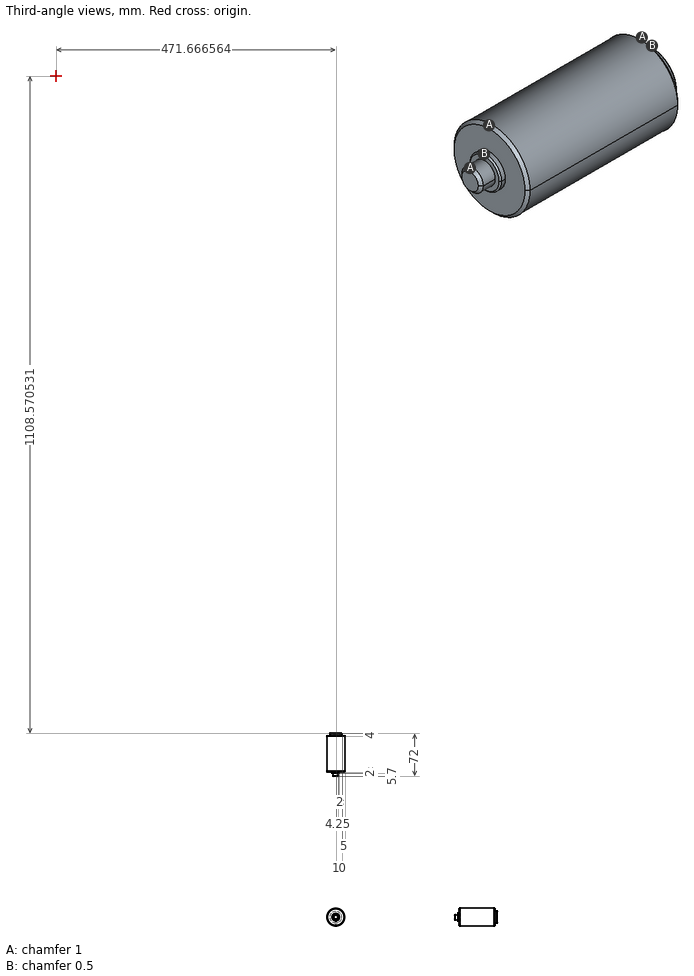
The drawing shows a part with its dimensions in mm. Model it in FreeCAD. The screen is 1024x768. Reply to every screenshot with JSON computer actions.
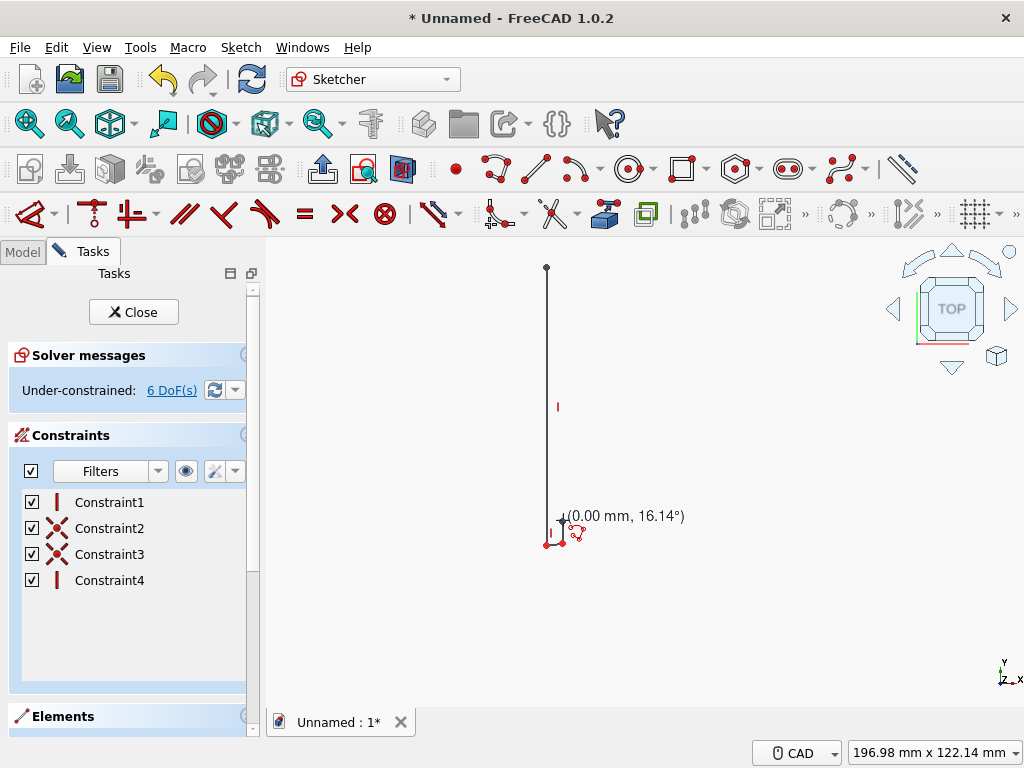
{"action": "scroll", "coordinate": [571, 520], "scroll_direction": "up", "scroll_amount": 4}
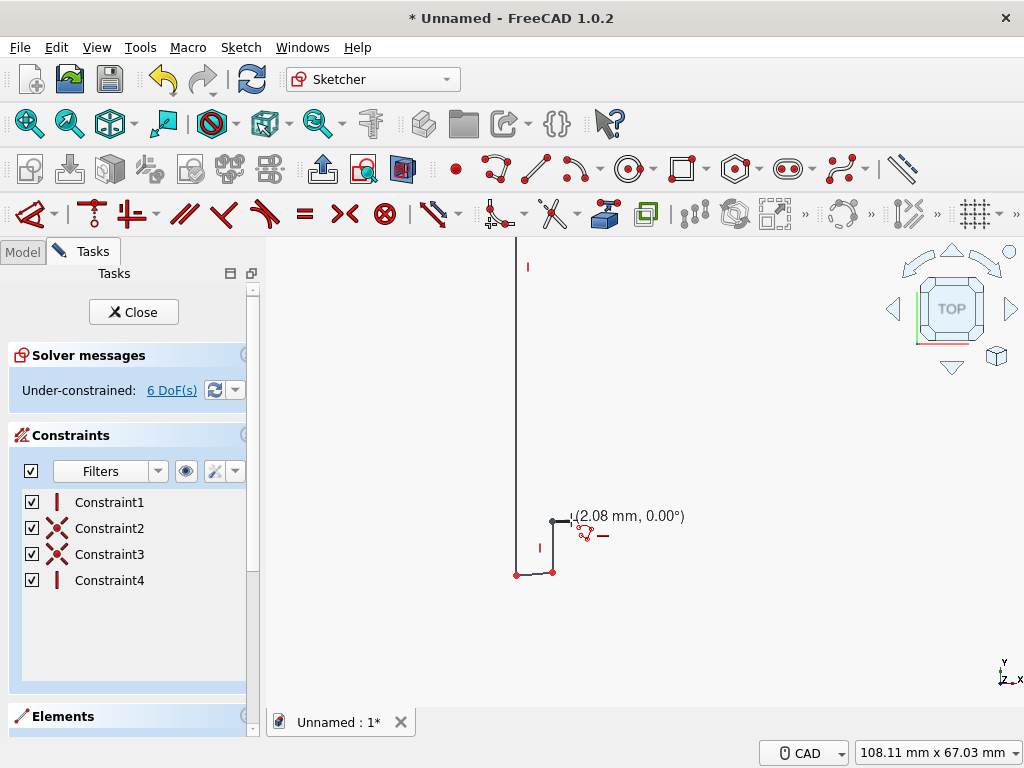
{"action": "left_click", "coordinate": [571, 519]}
{"action": "left_click", "coordinate": [571, 503]}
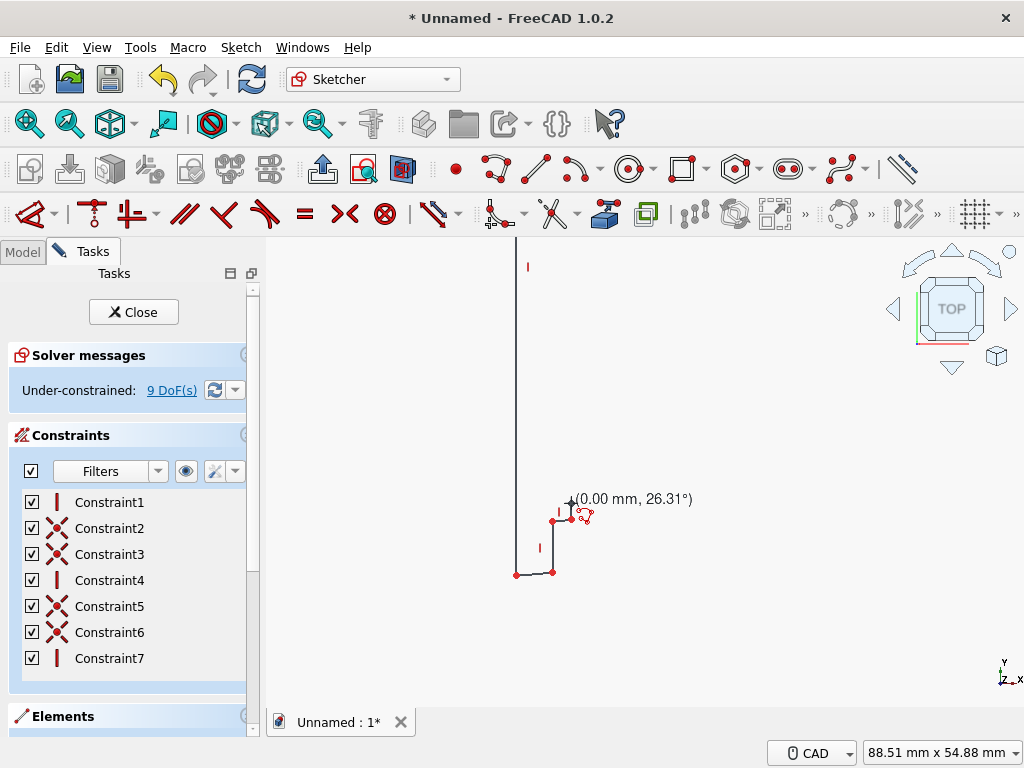
{"action": "scroll", "coordinate": [574, 667], "scroll_direction": "down", "scroll_amount": 5}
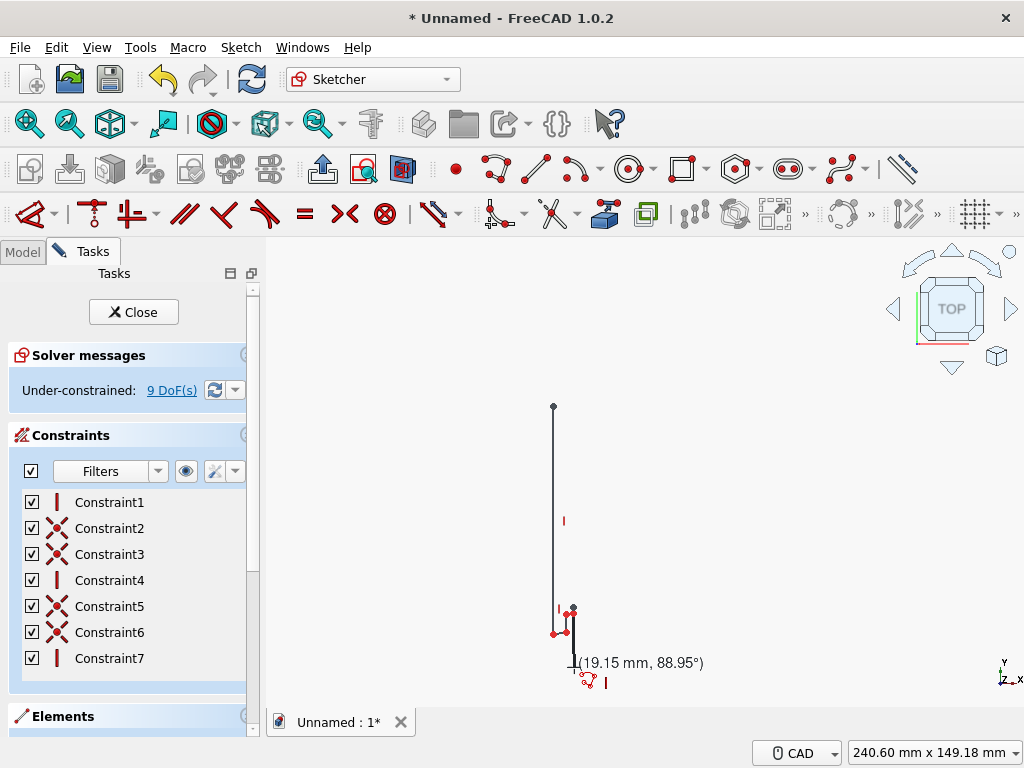
{"action": "left_click", "coordinate": [601, 607]}
{"action": "left_click", "coordinate": [601, 417]}
{"action": "left_click", "coordinate": [585, 417]}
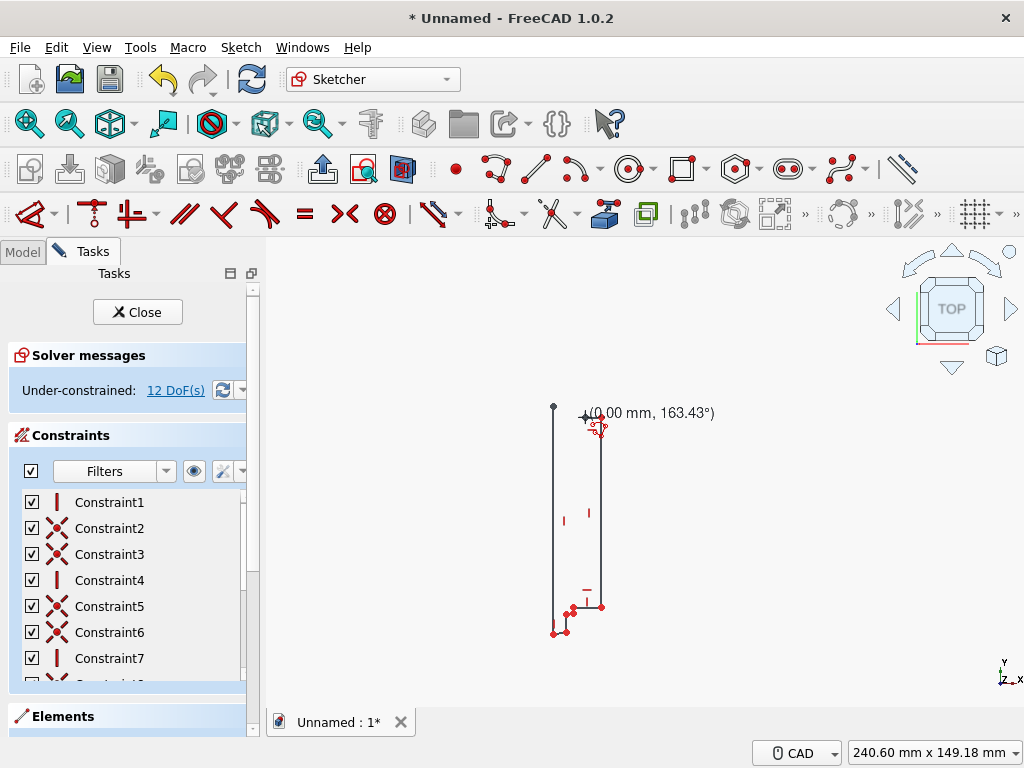
{"action": "scroll", "coordinate": [585, 405], "scroll_direction": "up", "scroll_amount": 2}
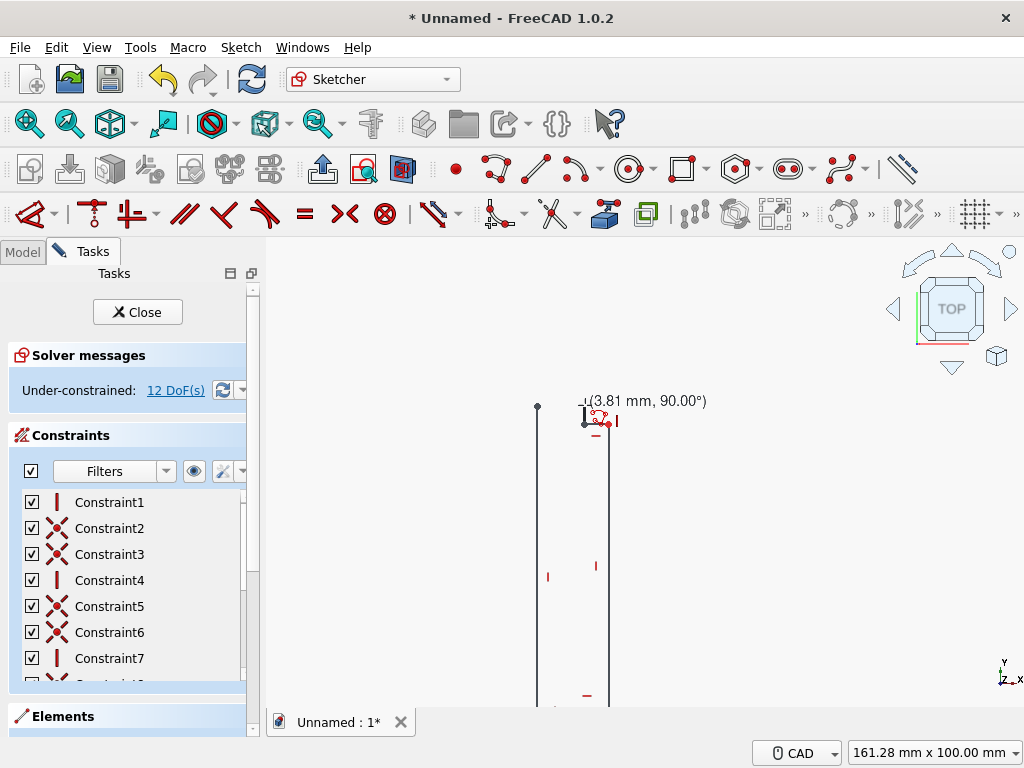
{"action": "left_click", "coordinate": [585, 404]}
{"action": "left_click", "coordinate": [537, 407]}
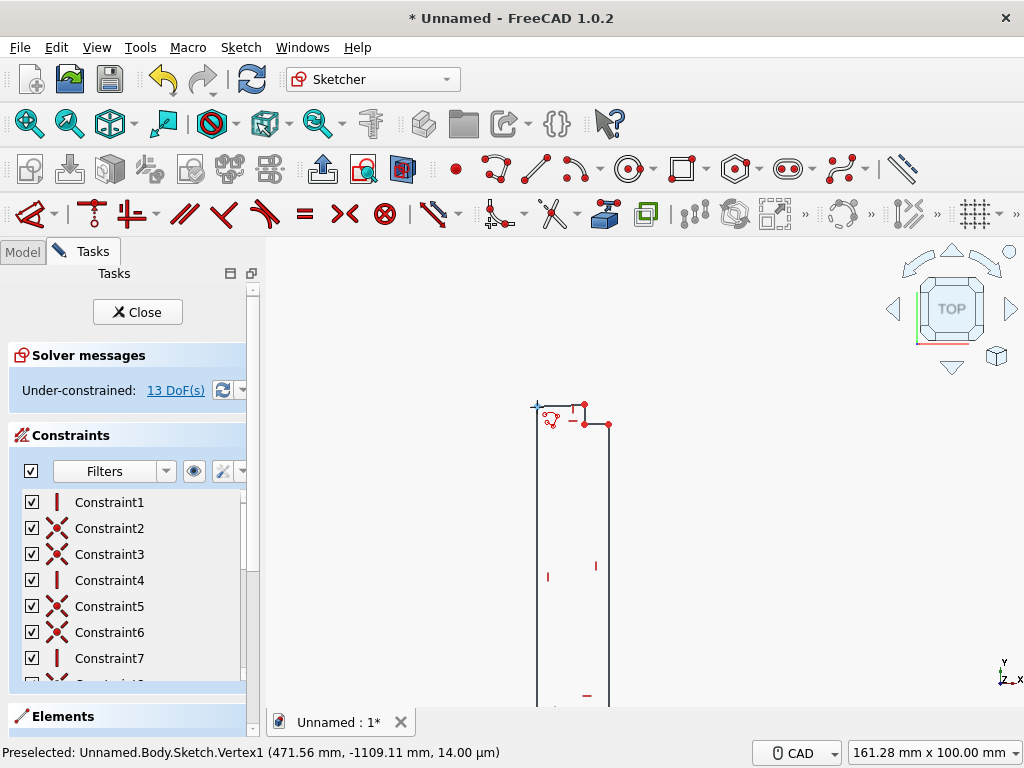
{"action": "key", "text": "g l"}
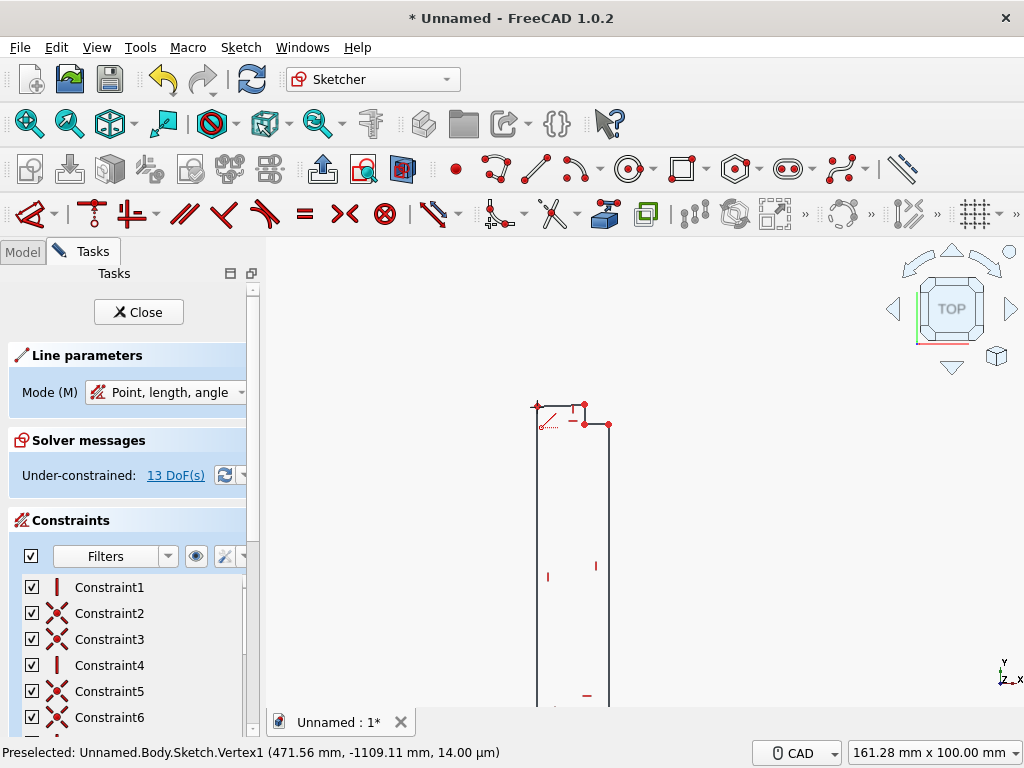
{"action": "left_click", "coordinate": [538, 370]}
{"action": "left_click", "coordinate": [538, 269]}
{"action": "key", "text": "Escape"}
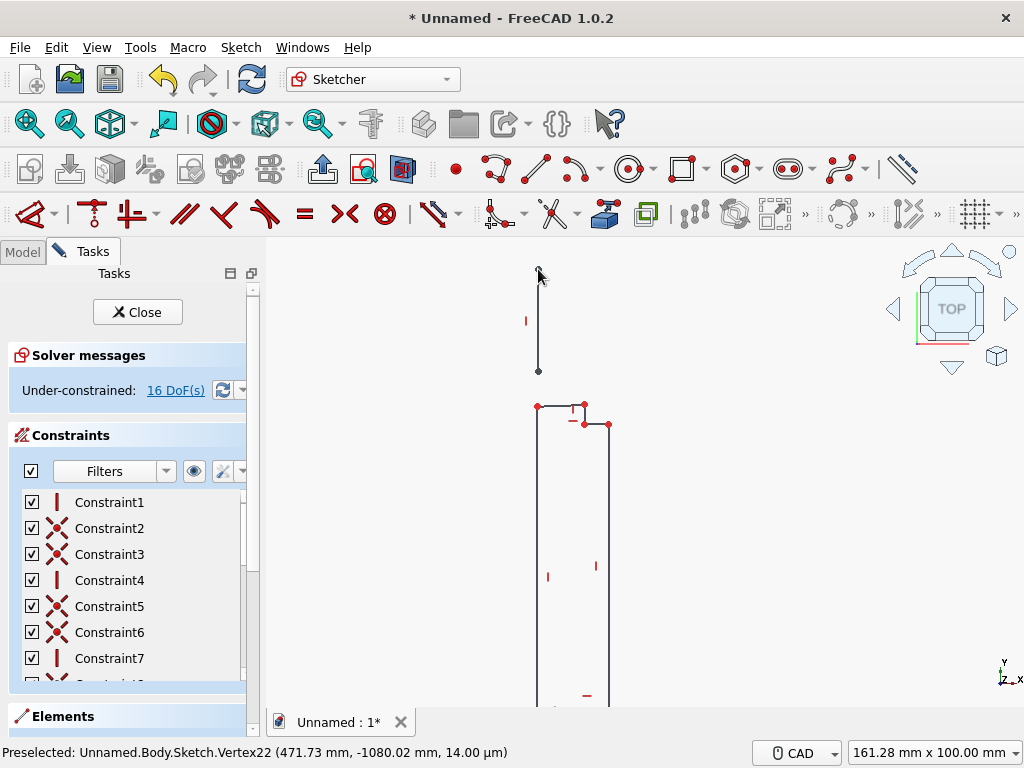
{"action": "left_click", "coordinate": [538, 341]}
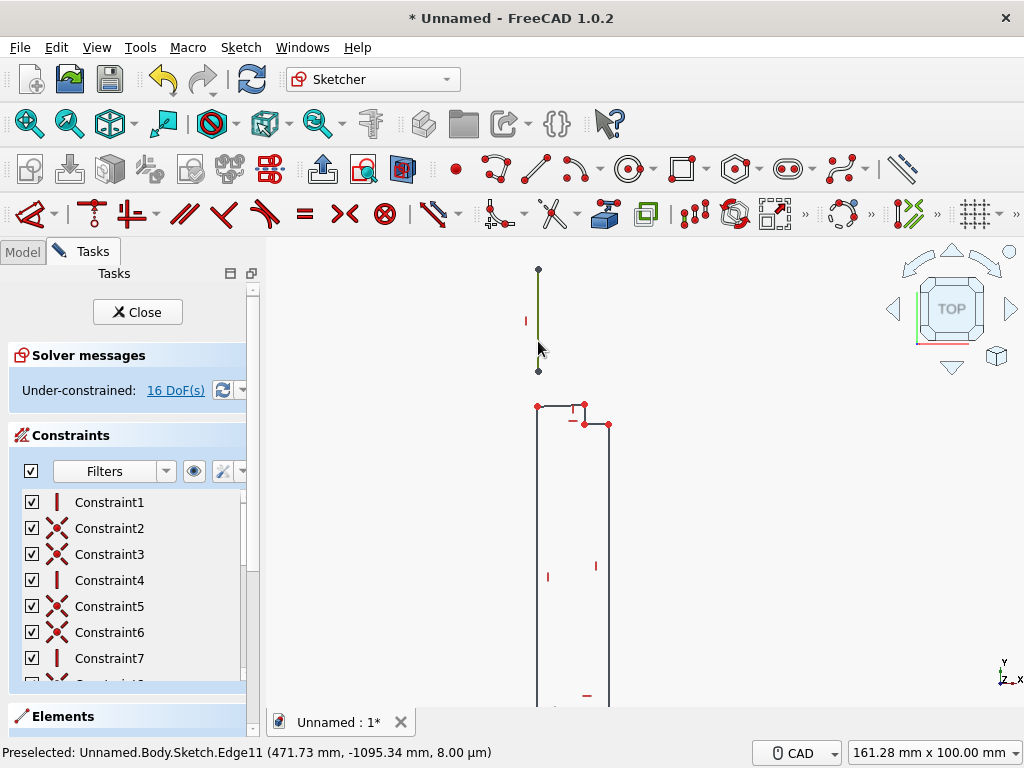
{"action": "key", "text": "g n"}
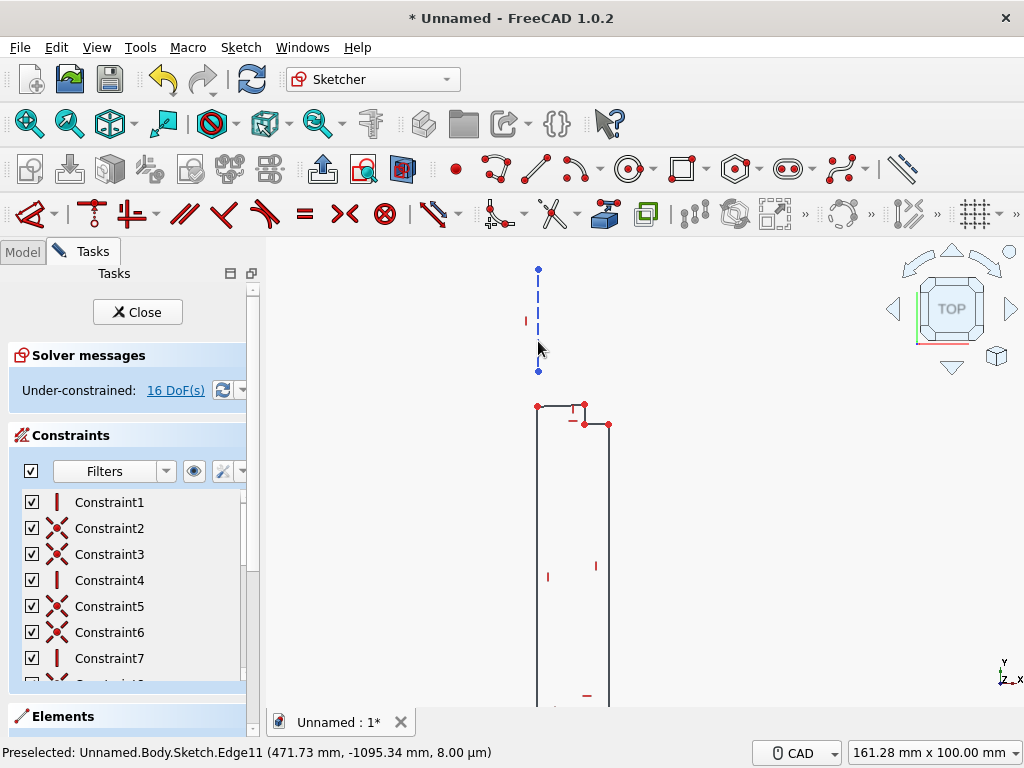
{"action": "scroll", "coordinate": [584, 403], "scroll_direction": "down", "scroll_amount": 2}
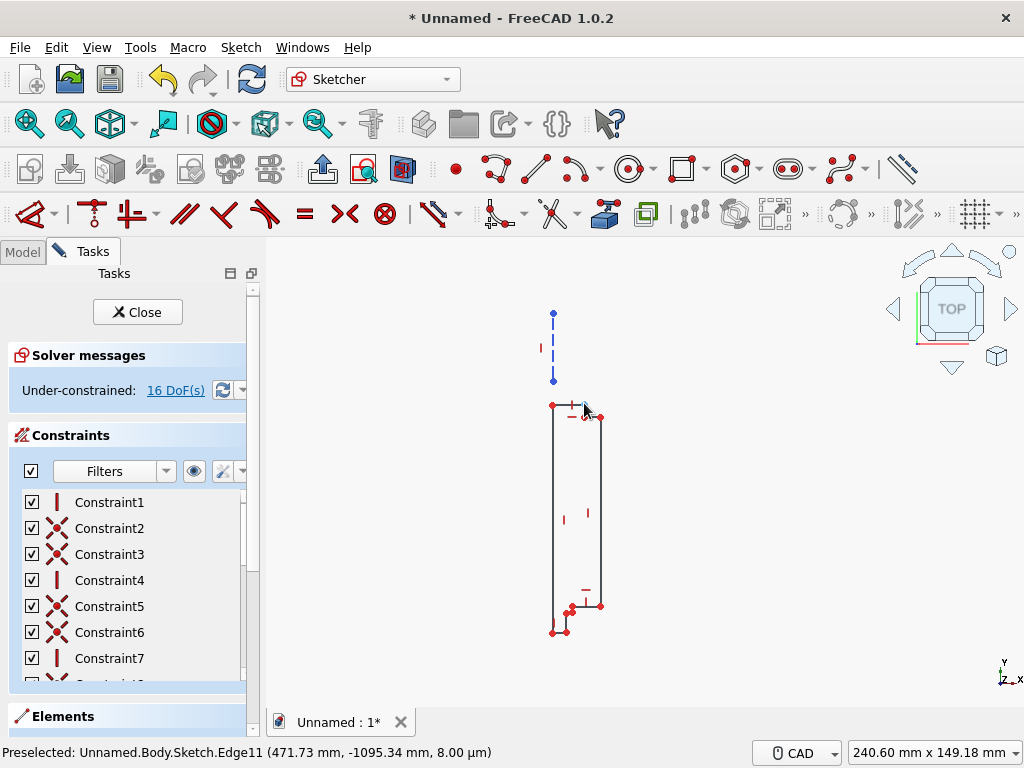
{"action": "scroll", "coordinate": [559, 633], "scroll_direction": "up", "scroll_amount": 4}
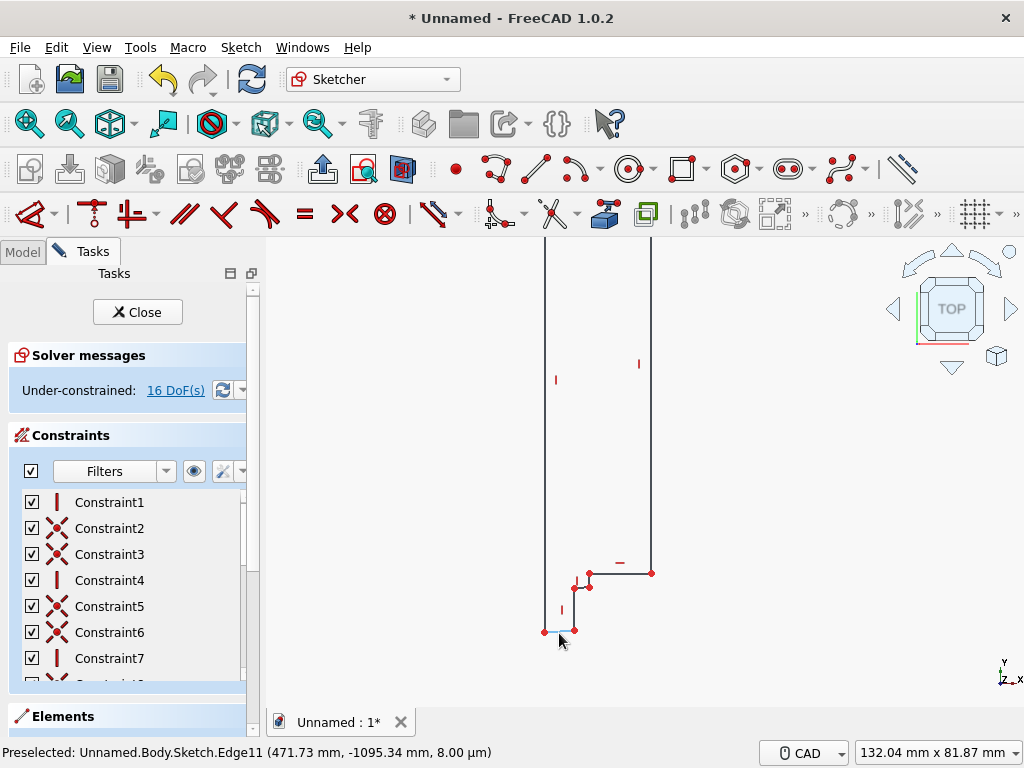
{"action": "left_click", "coordinate": [559, 632]}